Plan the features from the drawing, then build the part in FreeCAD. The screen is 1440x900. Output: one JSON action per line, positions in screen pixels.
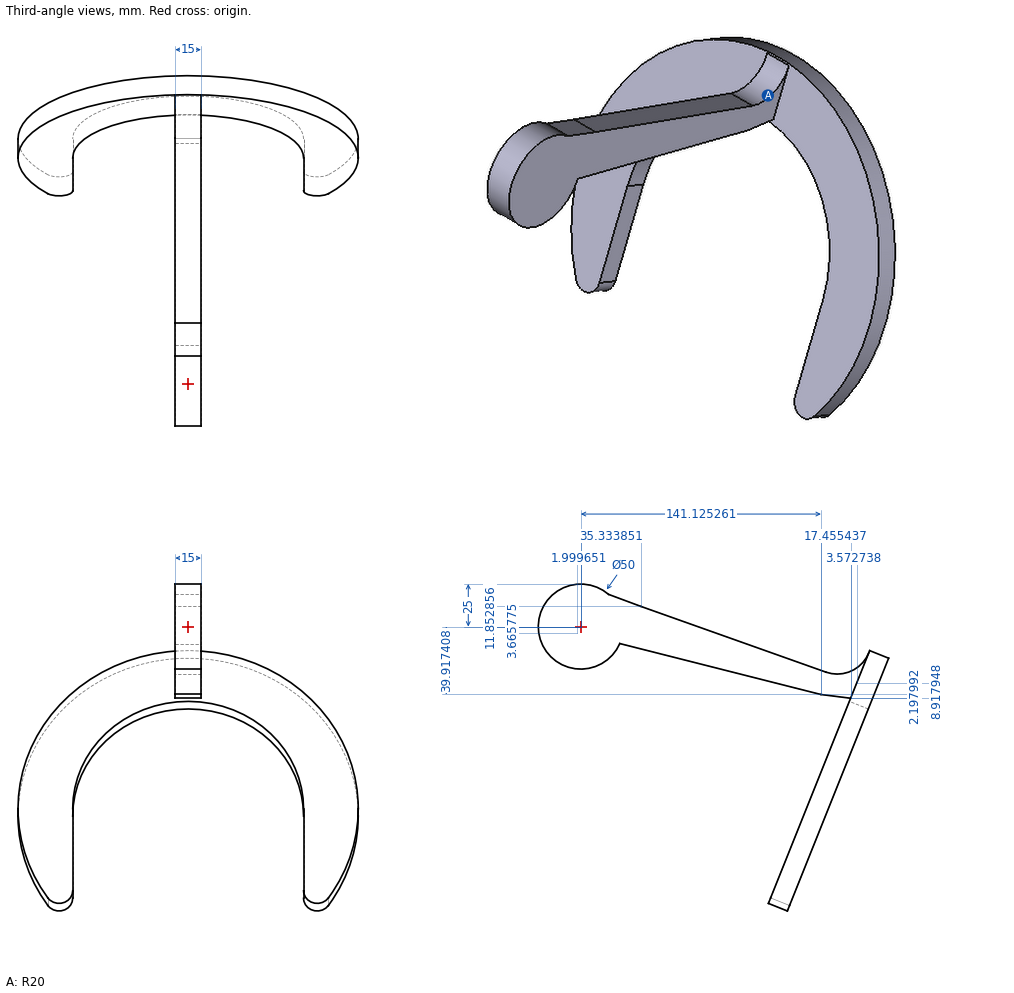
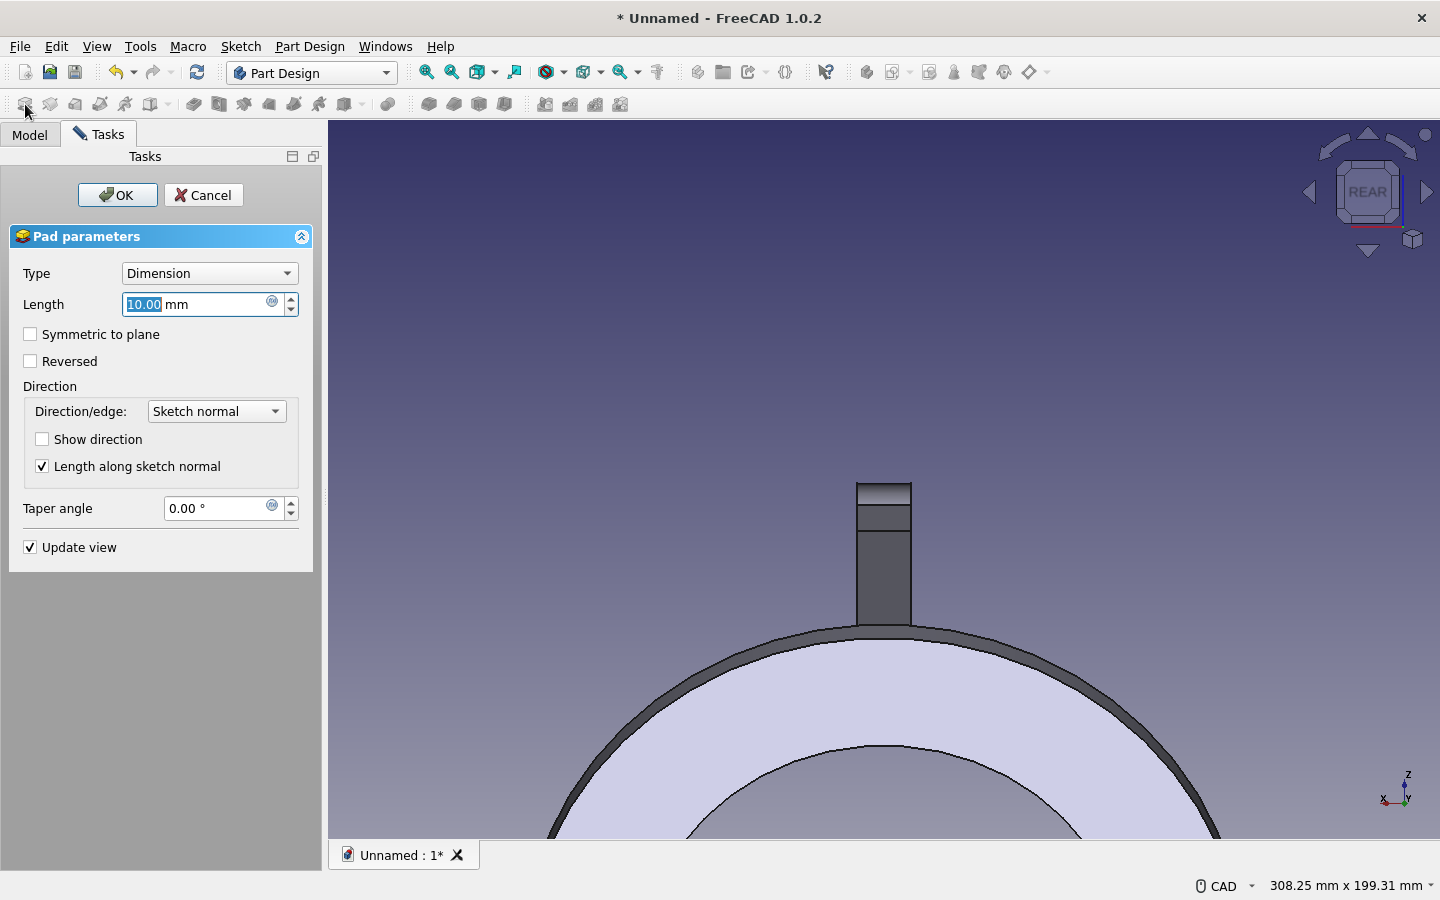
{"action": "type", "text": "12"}
{"action": "key", "text": "Tab"}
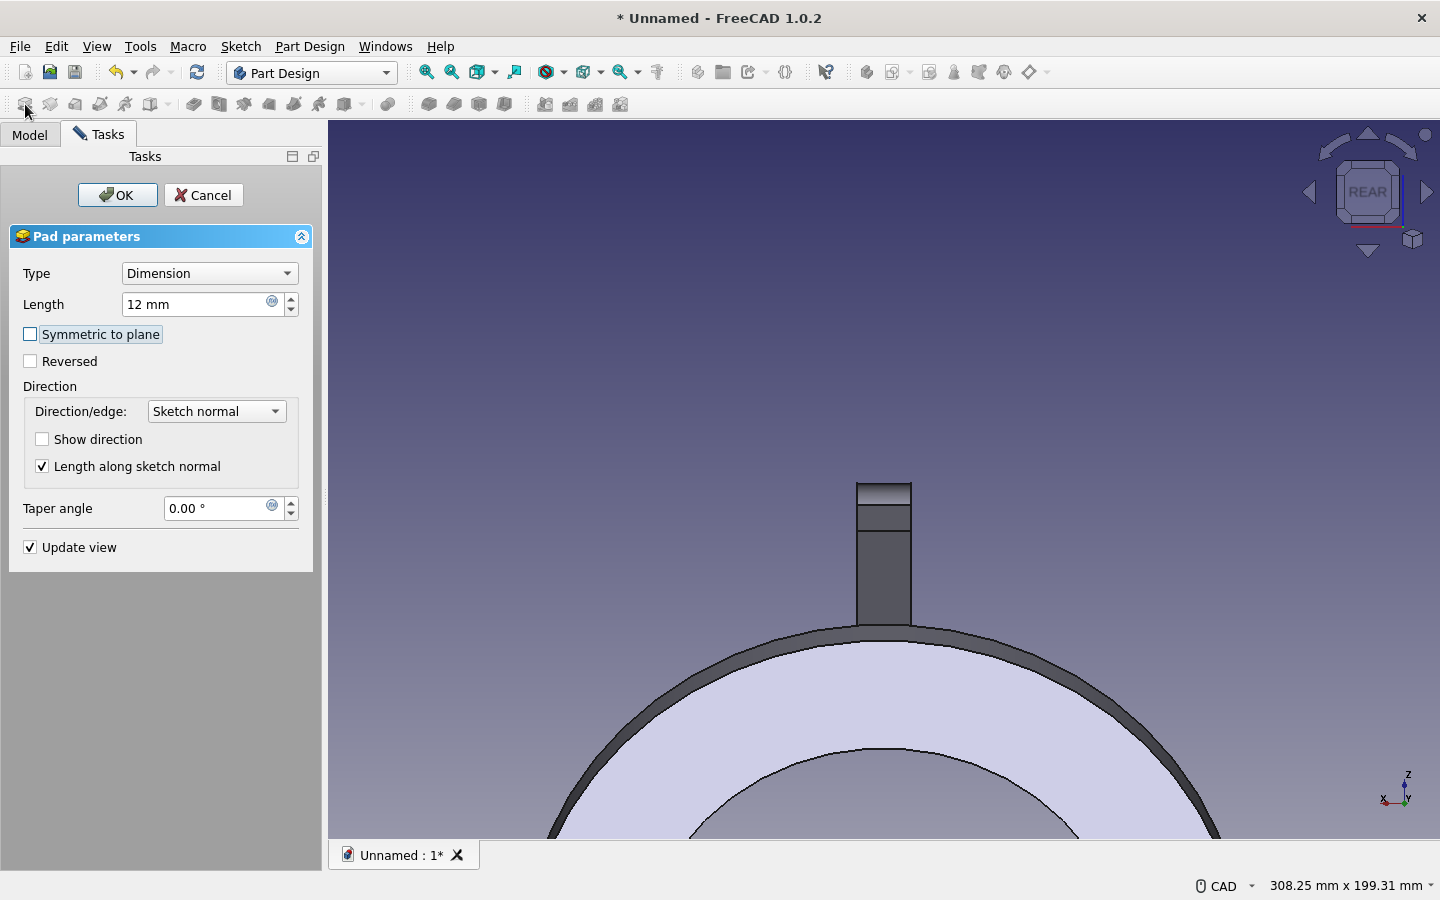
{"action": "left_click", "coordinate": [118, 195]}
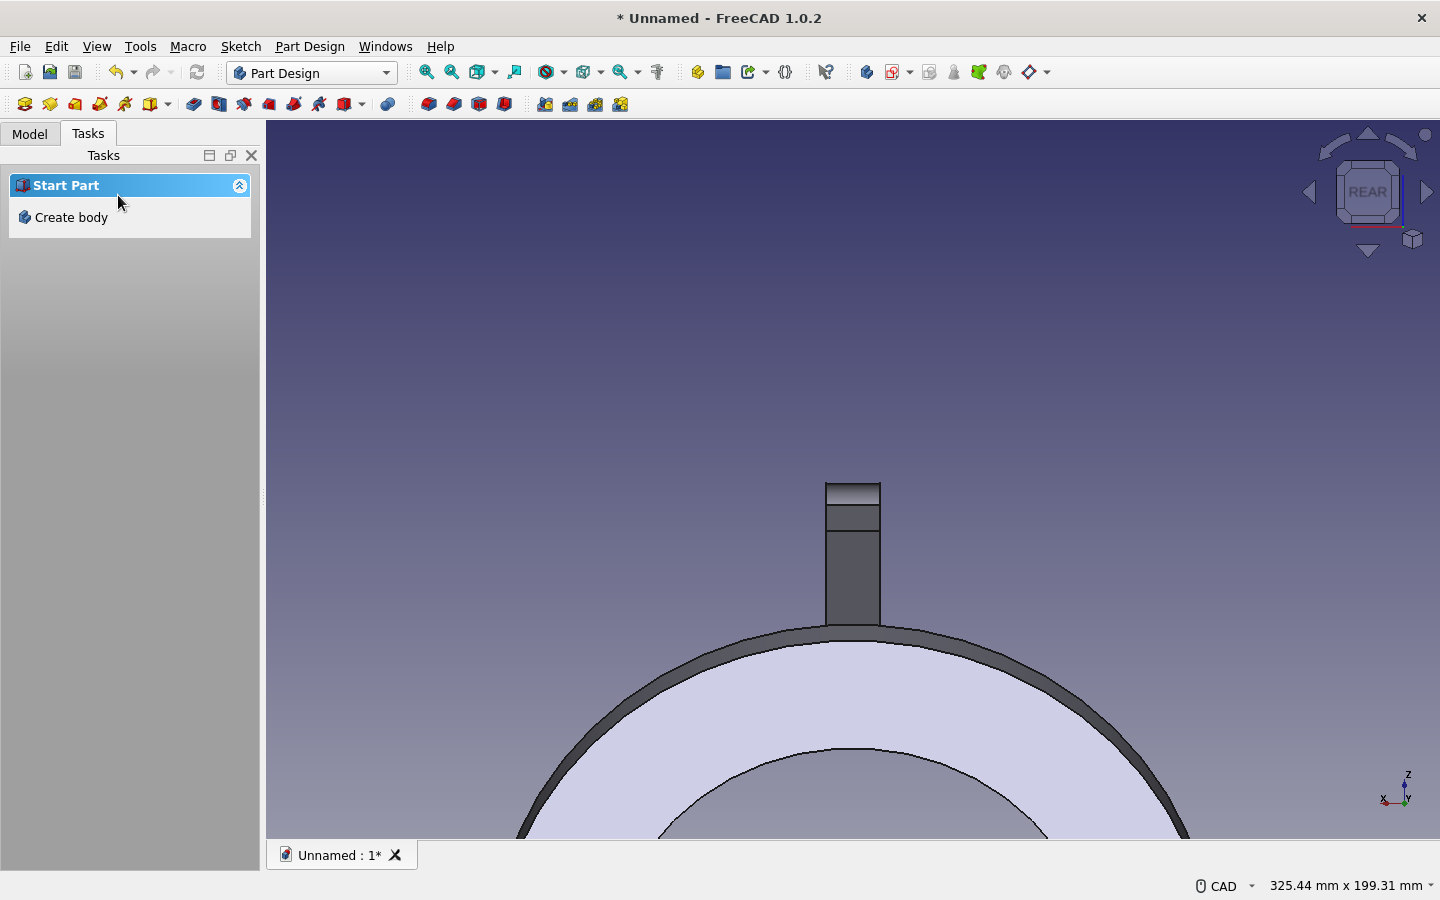
{"action": "left_click", "coordinate": [427, 72]}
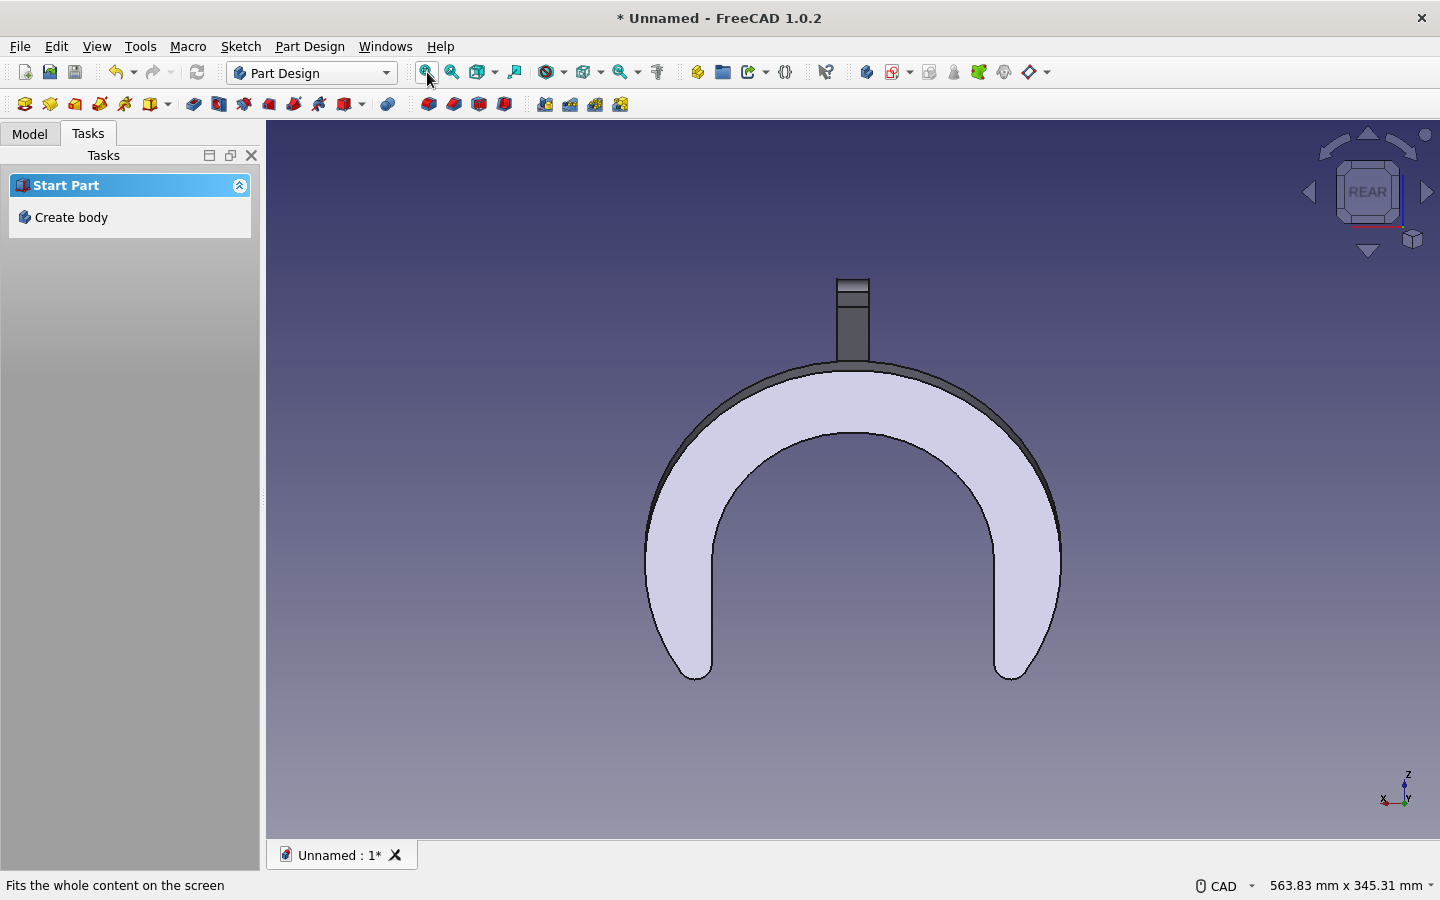
{"action": "key", "text": "0"}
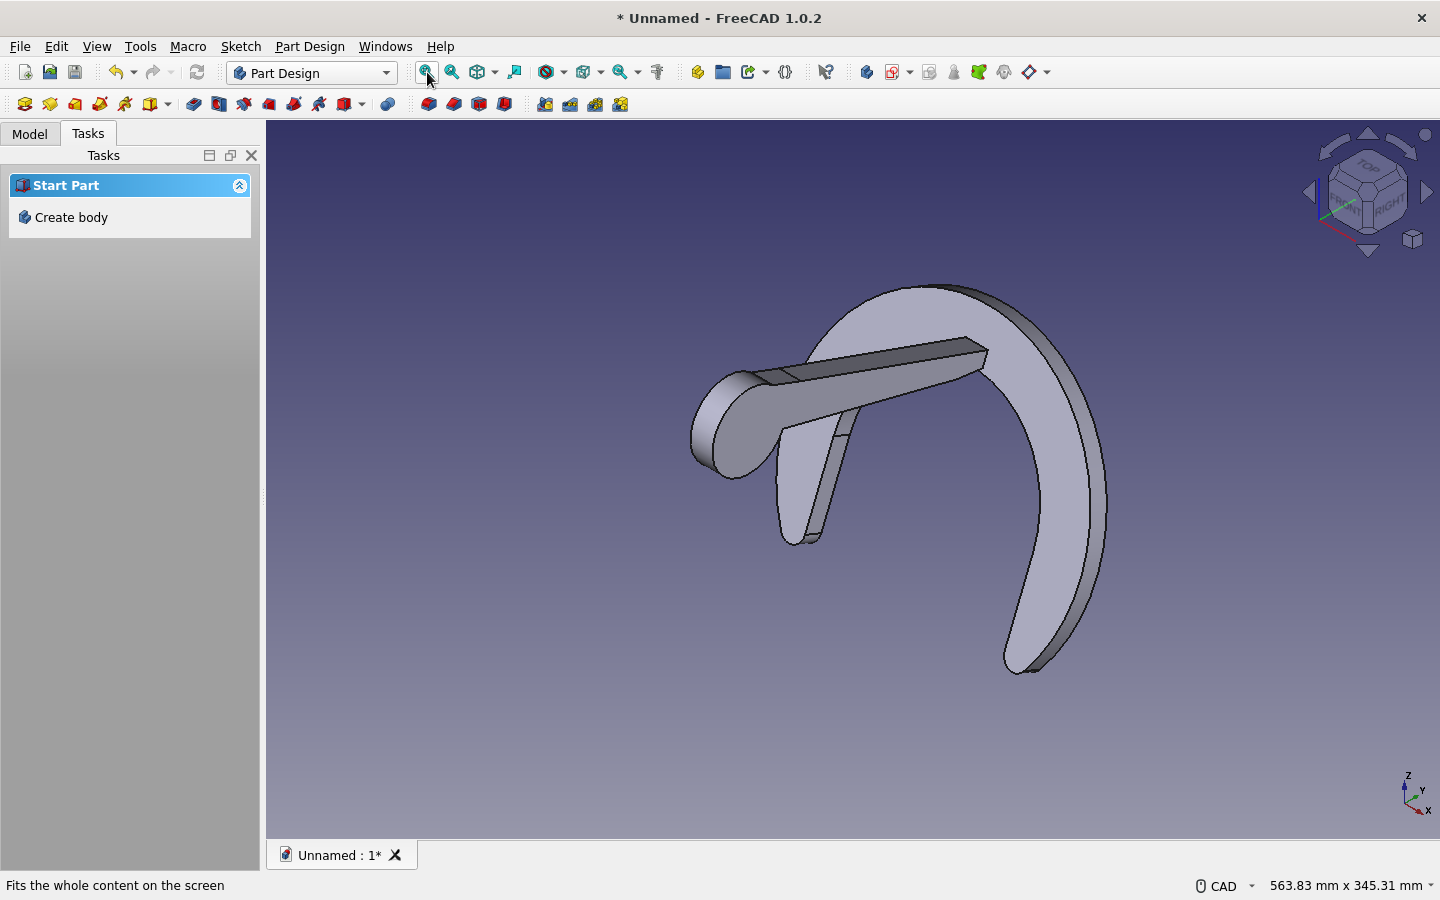
{"action": "key", "text": "2"}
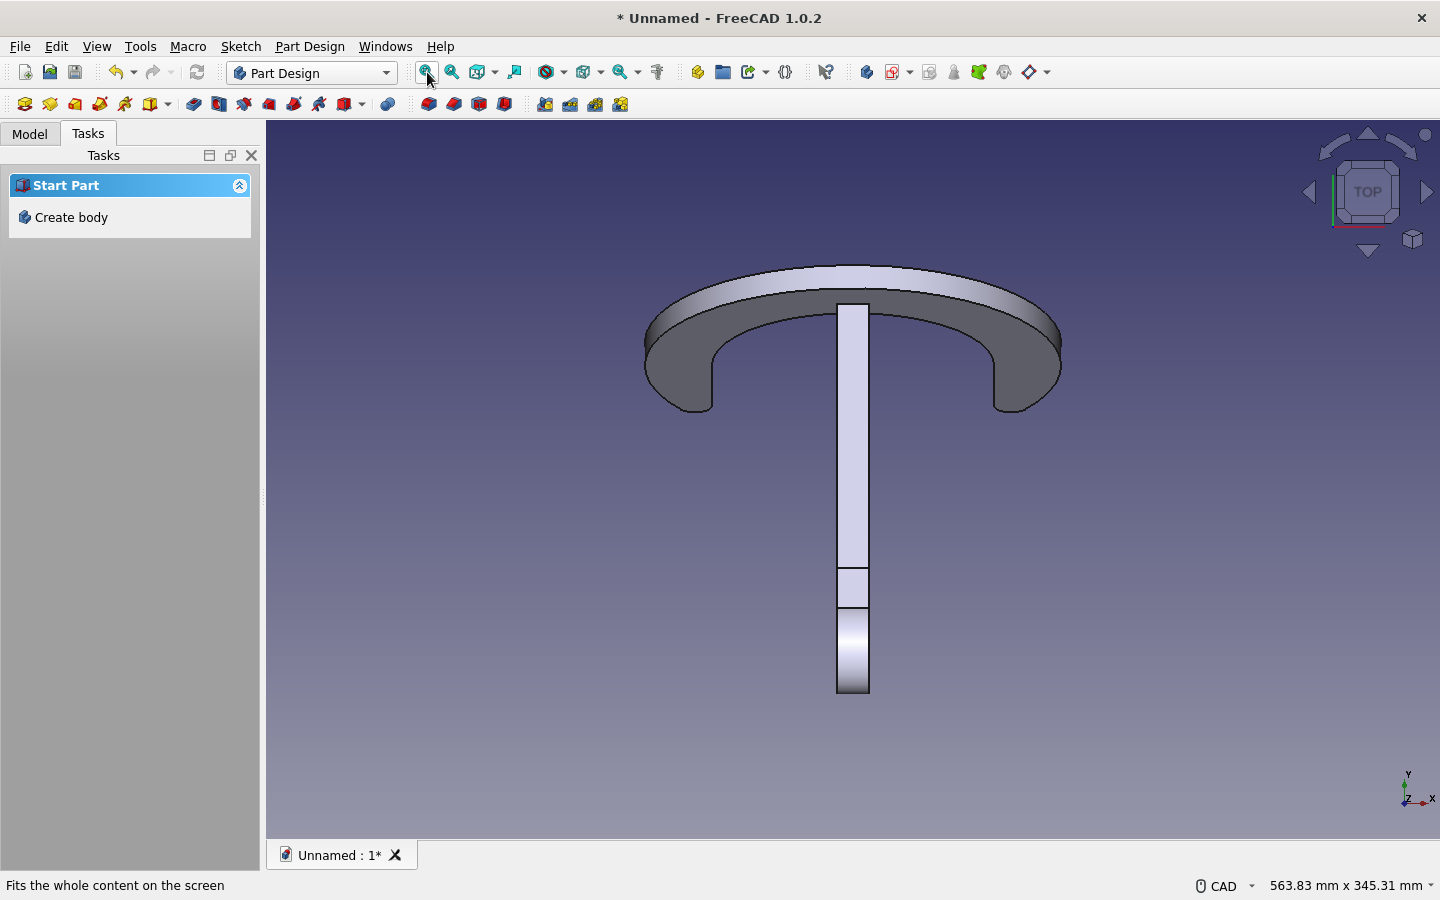
{"action": "key", "text": "1"}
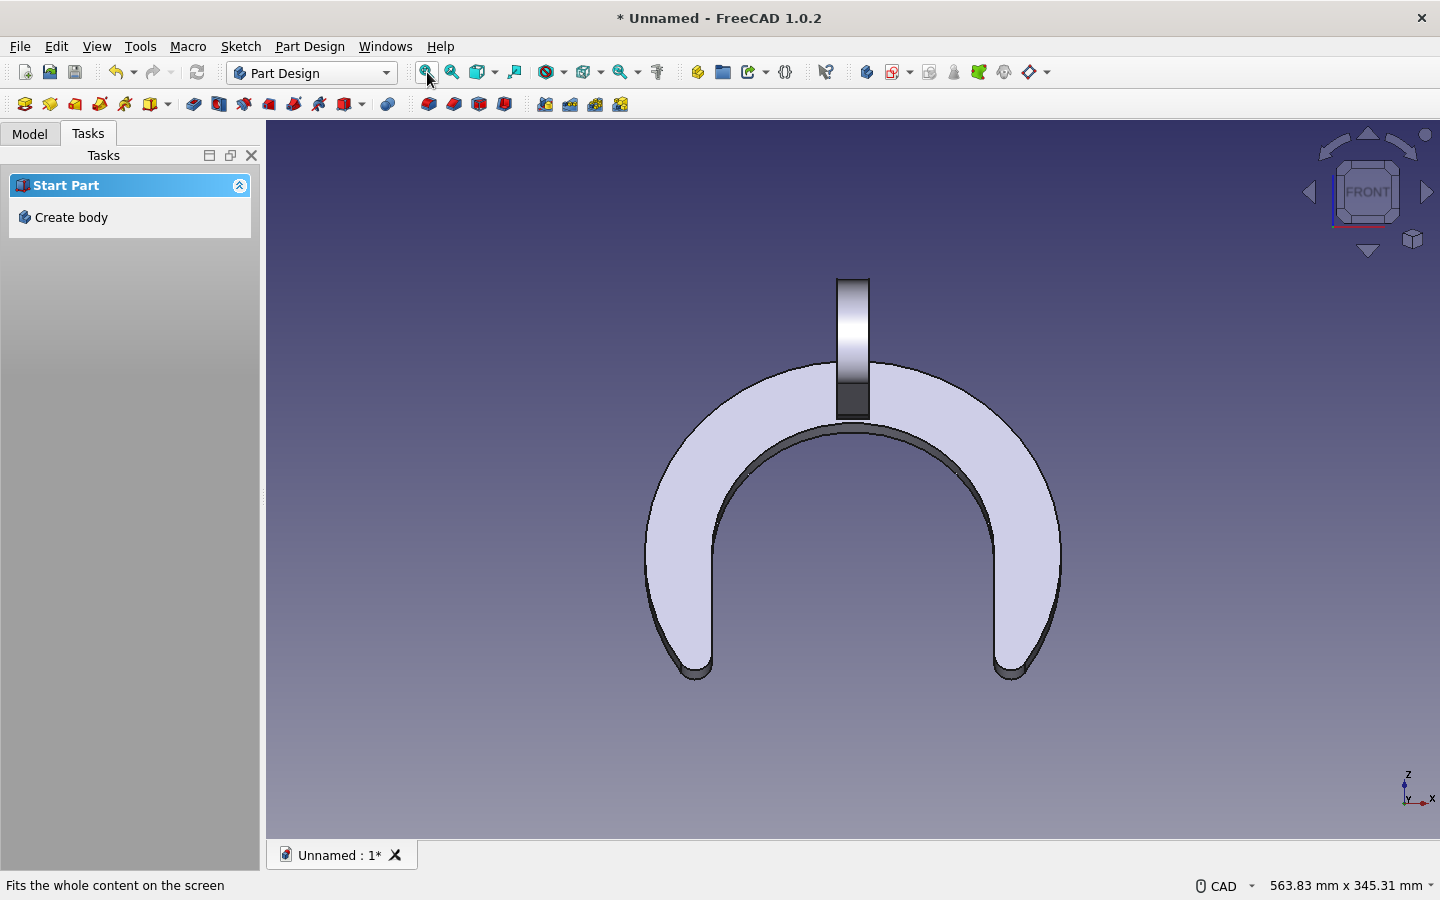
{"action": "key", "text": "3"}